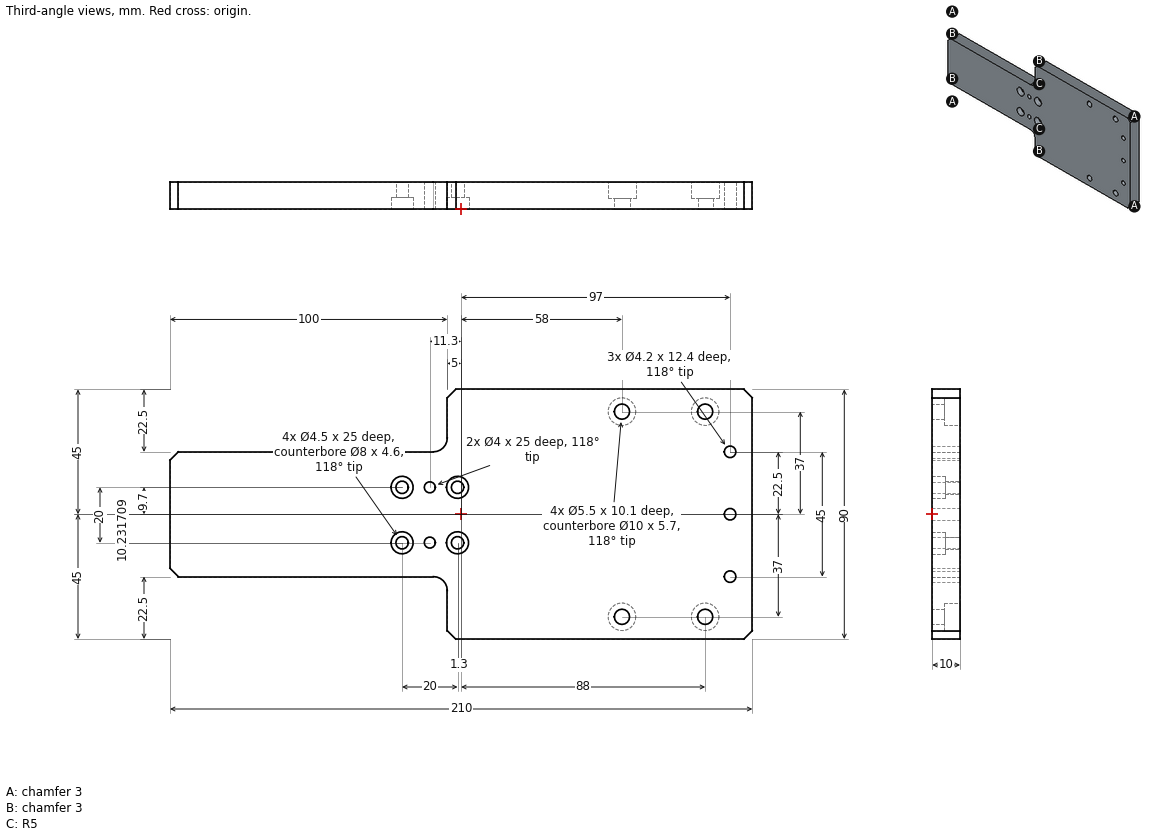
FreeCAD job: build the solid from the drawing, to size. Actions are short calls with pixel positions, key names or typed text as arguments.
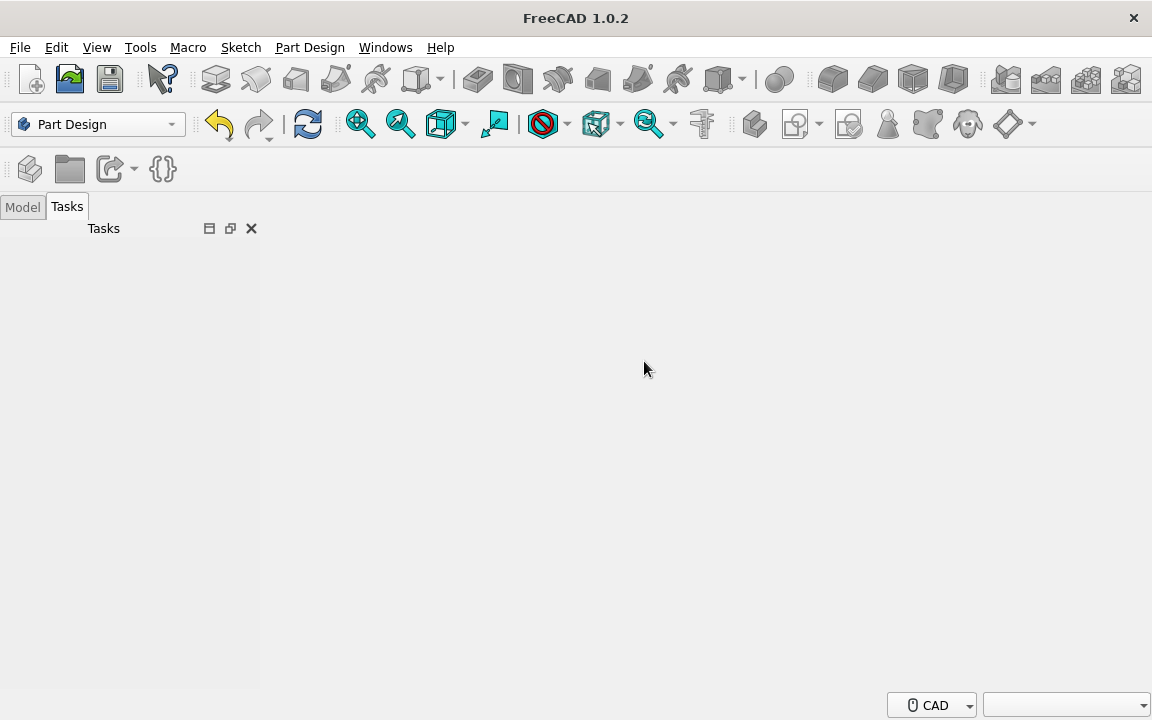
click(30, 80)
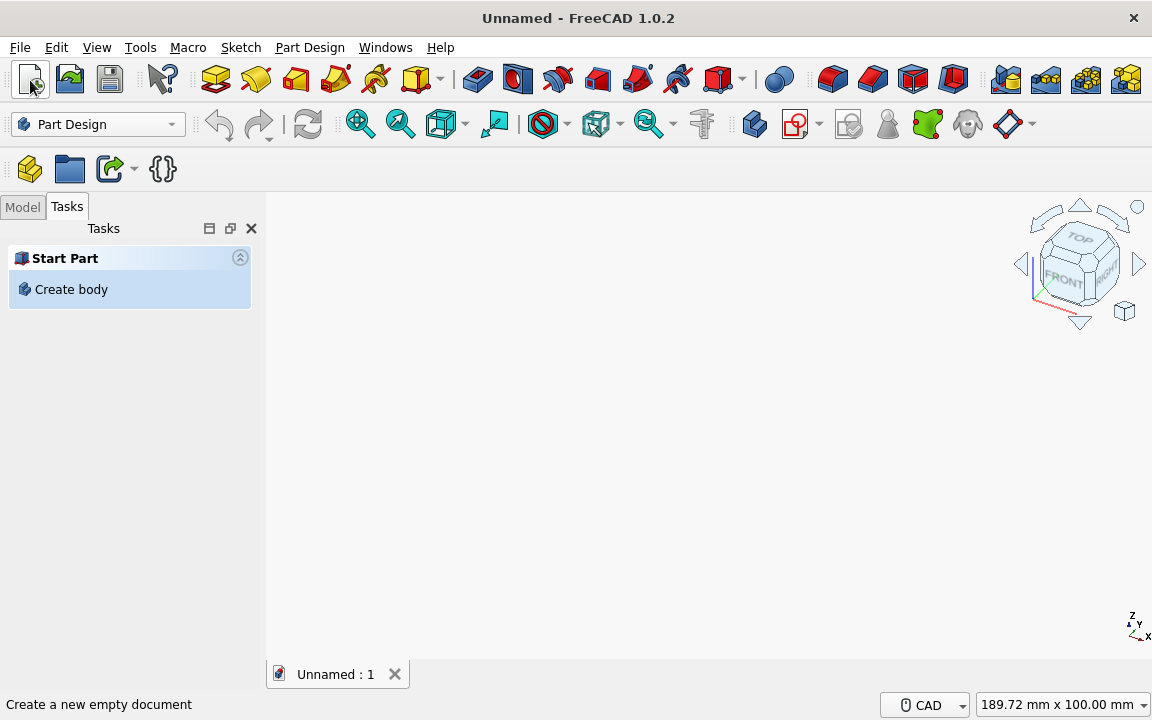
click(796, 124)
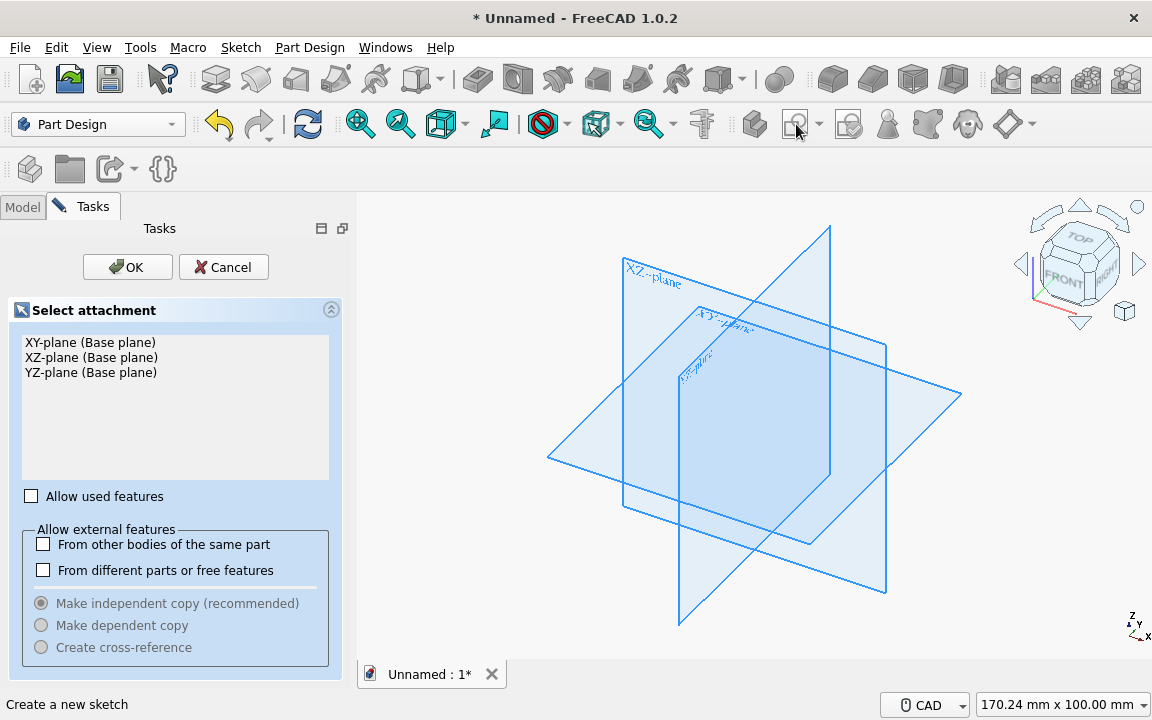
click(82, 358)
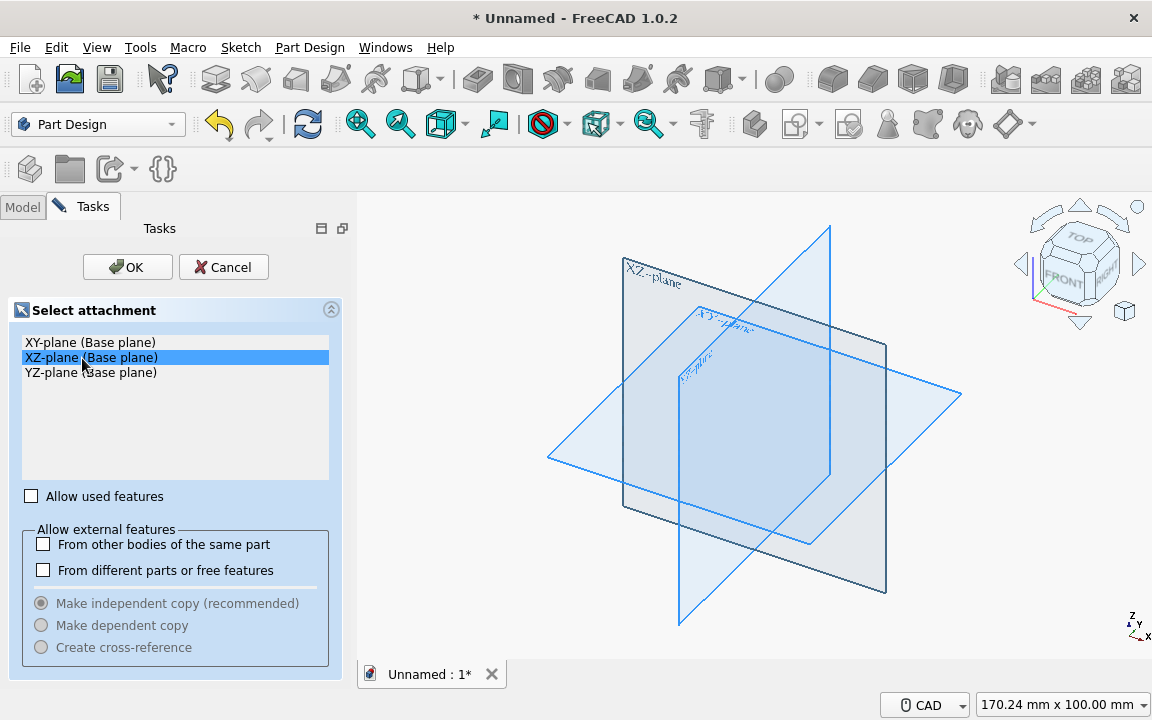
click(128, 267)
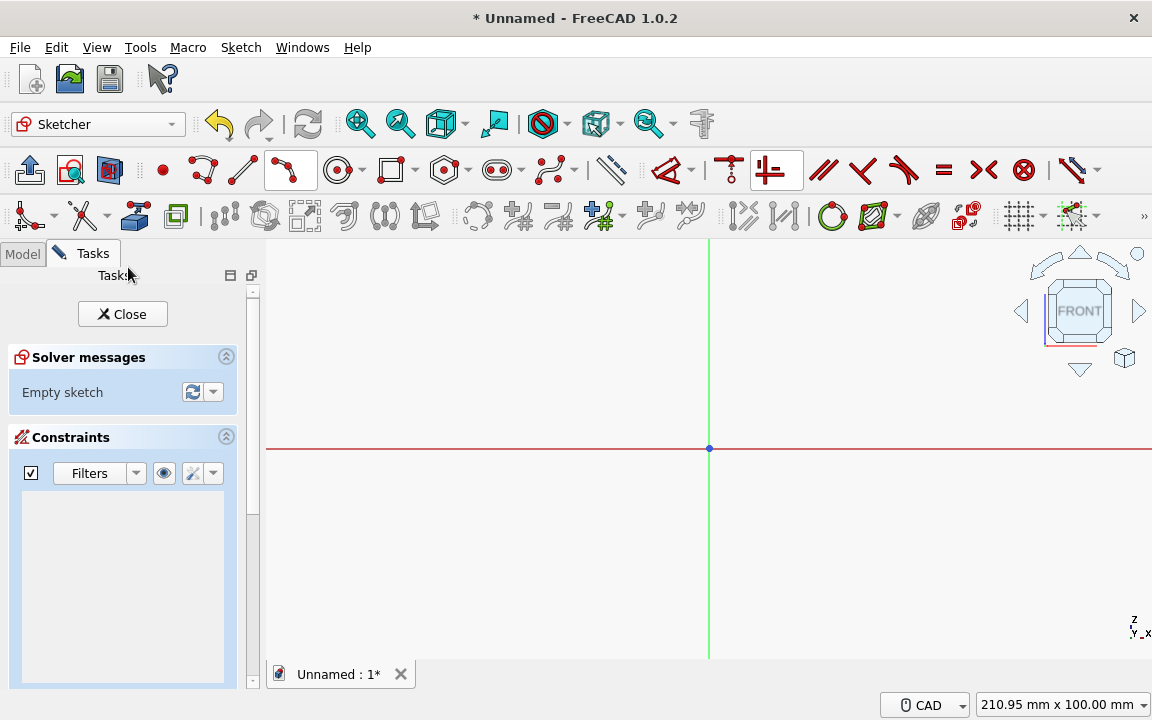
scroll(557, 449, down, 3)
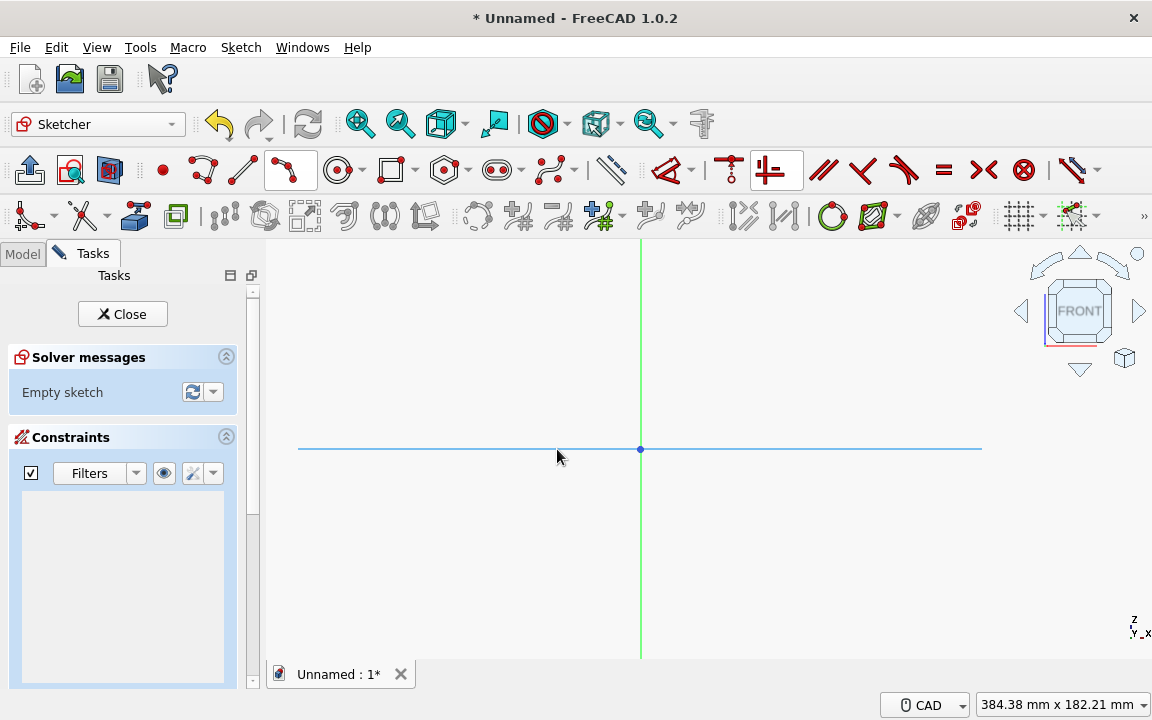
click(418, 170)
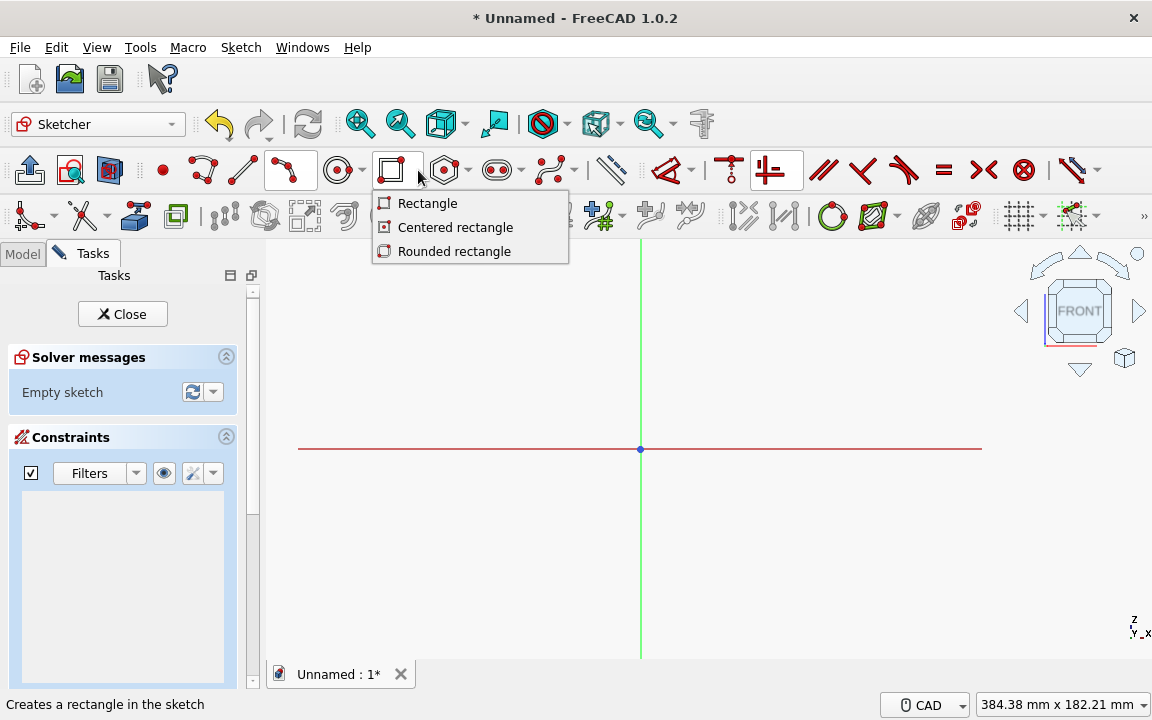
click(470, 227)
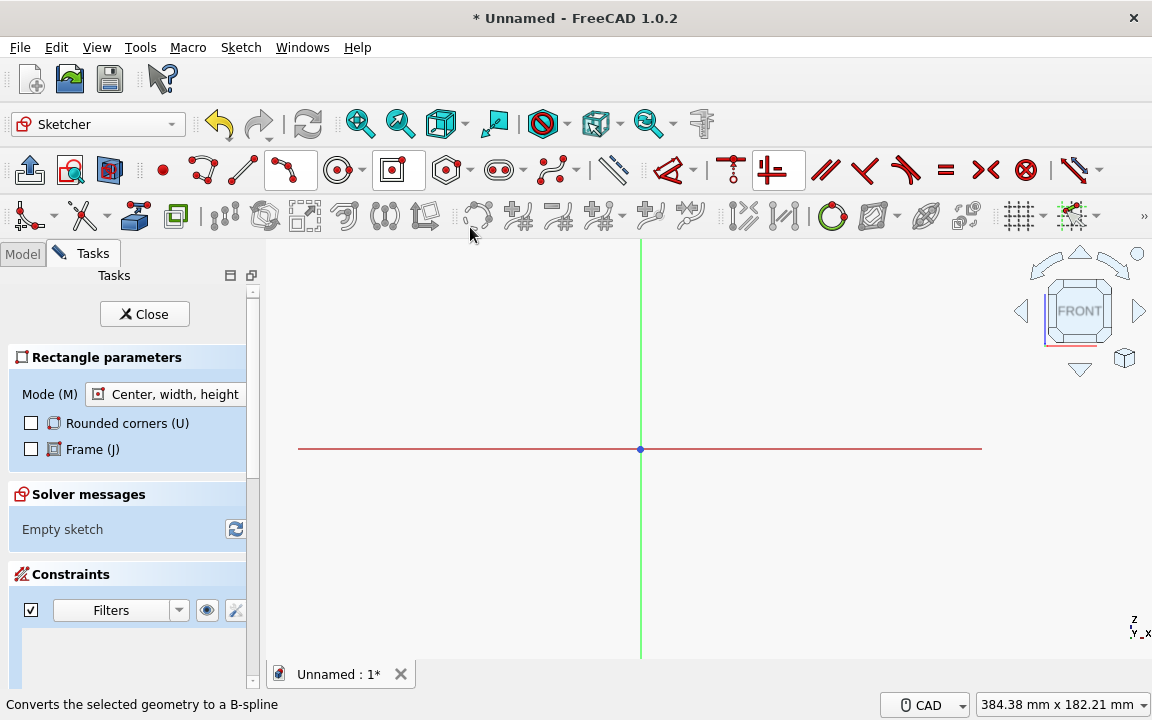
click(641, 449)
click(883, 346)
key(Escape)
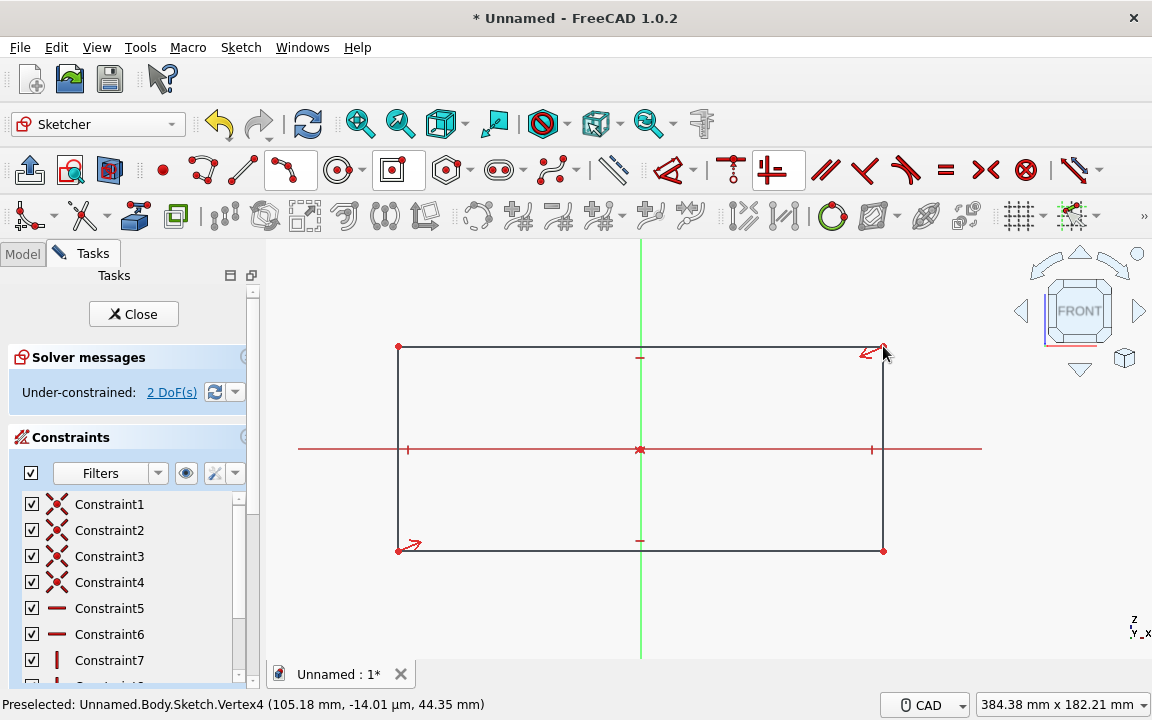
click(883, 490)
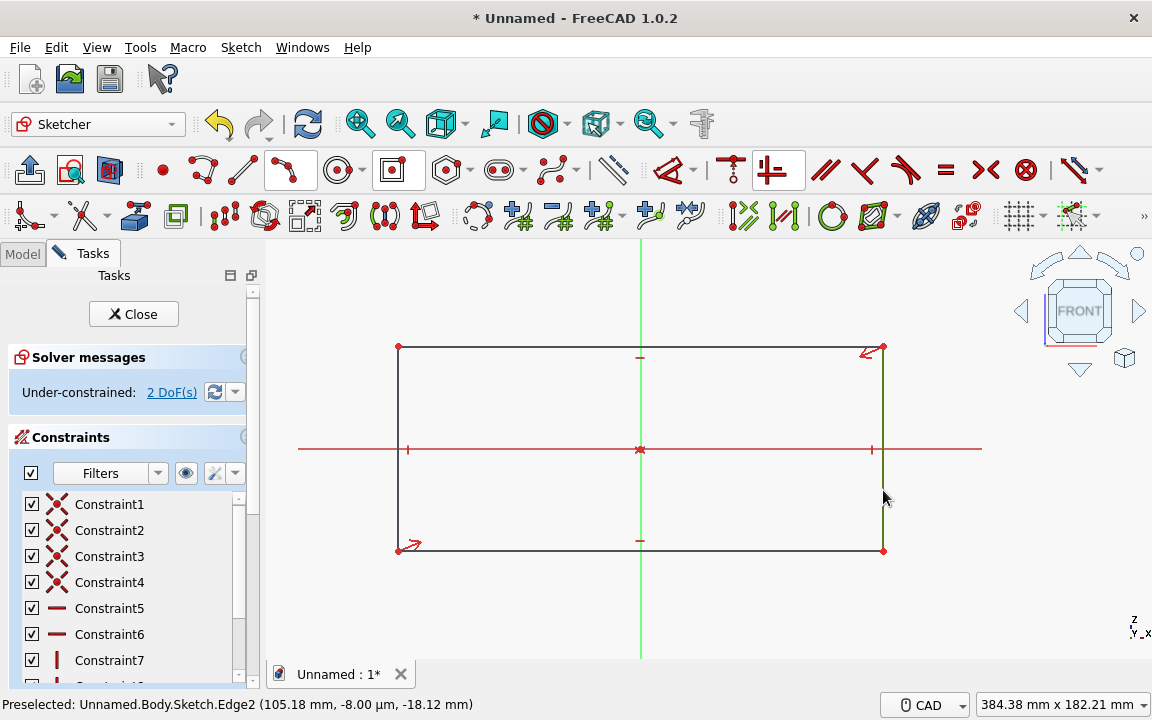
click(696, 170)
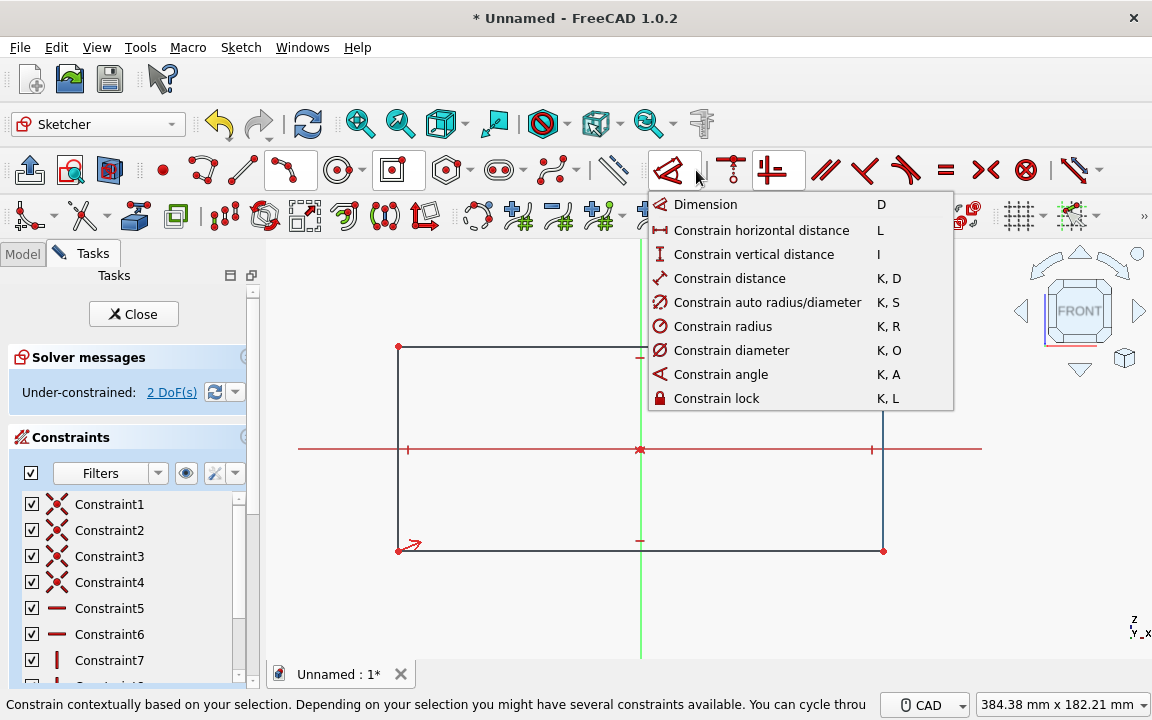
click(801, 254)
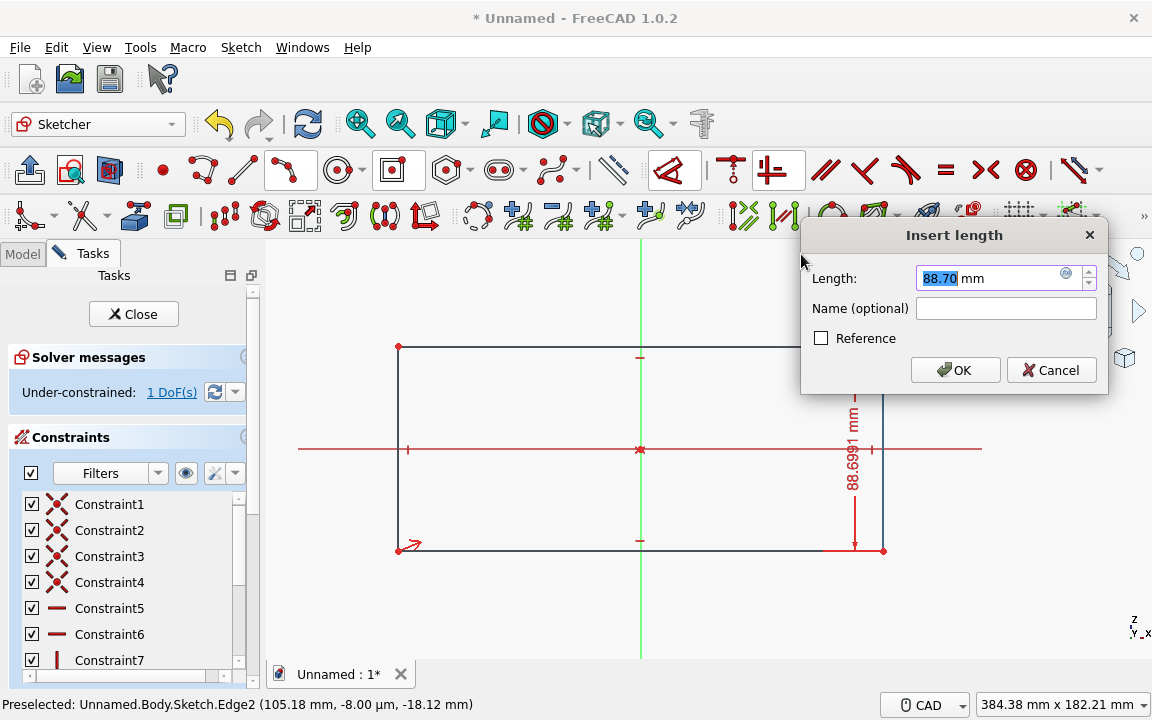
text(90)
key(Return)